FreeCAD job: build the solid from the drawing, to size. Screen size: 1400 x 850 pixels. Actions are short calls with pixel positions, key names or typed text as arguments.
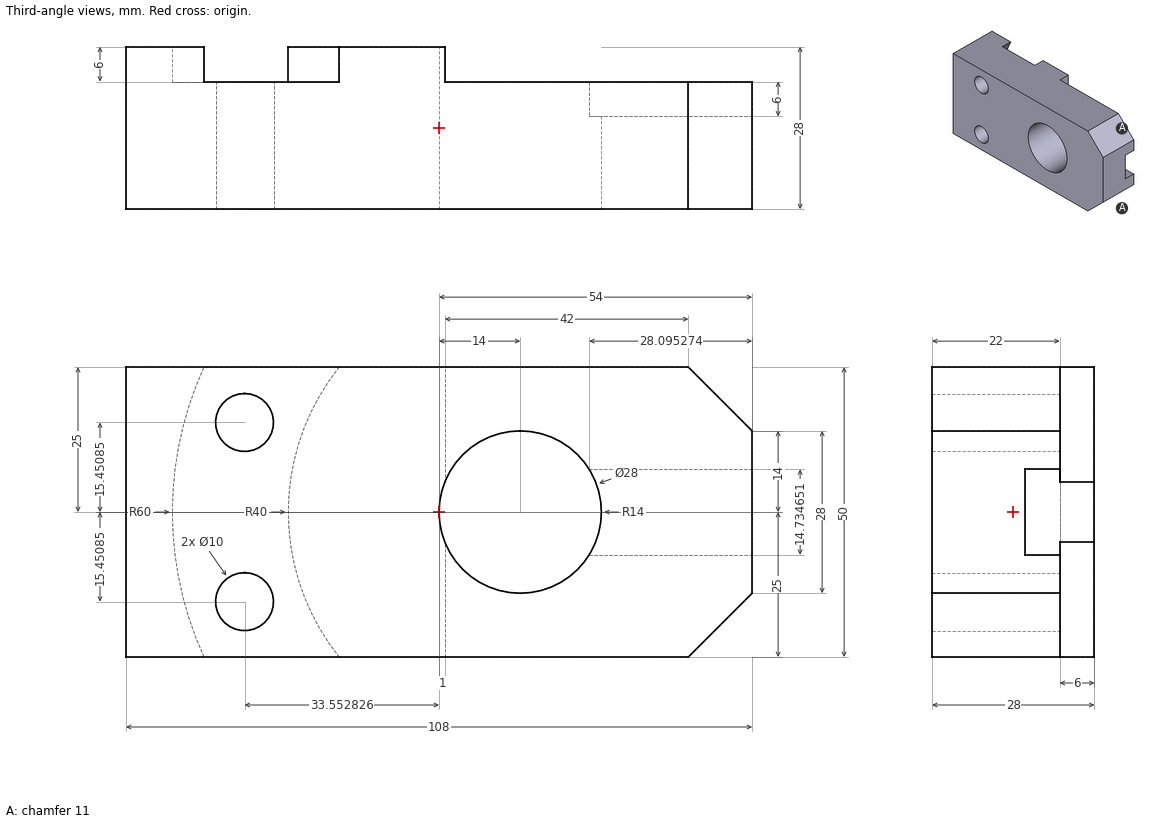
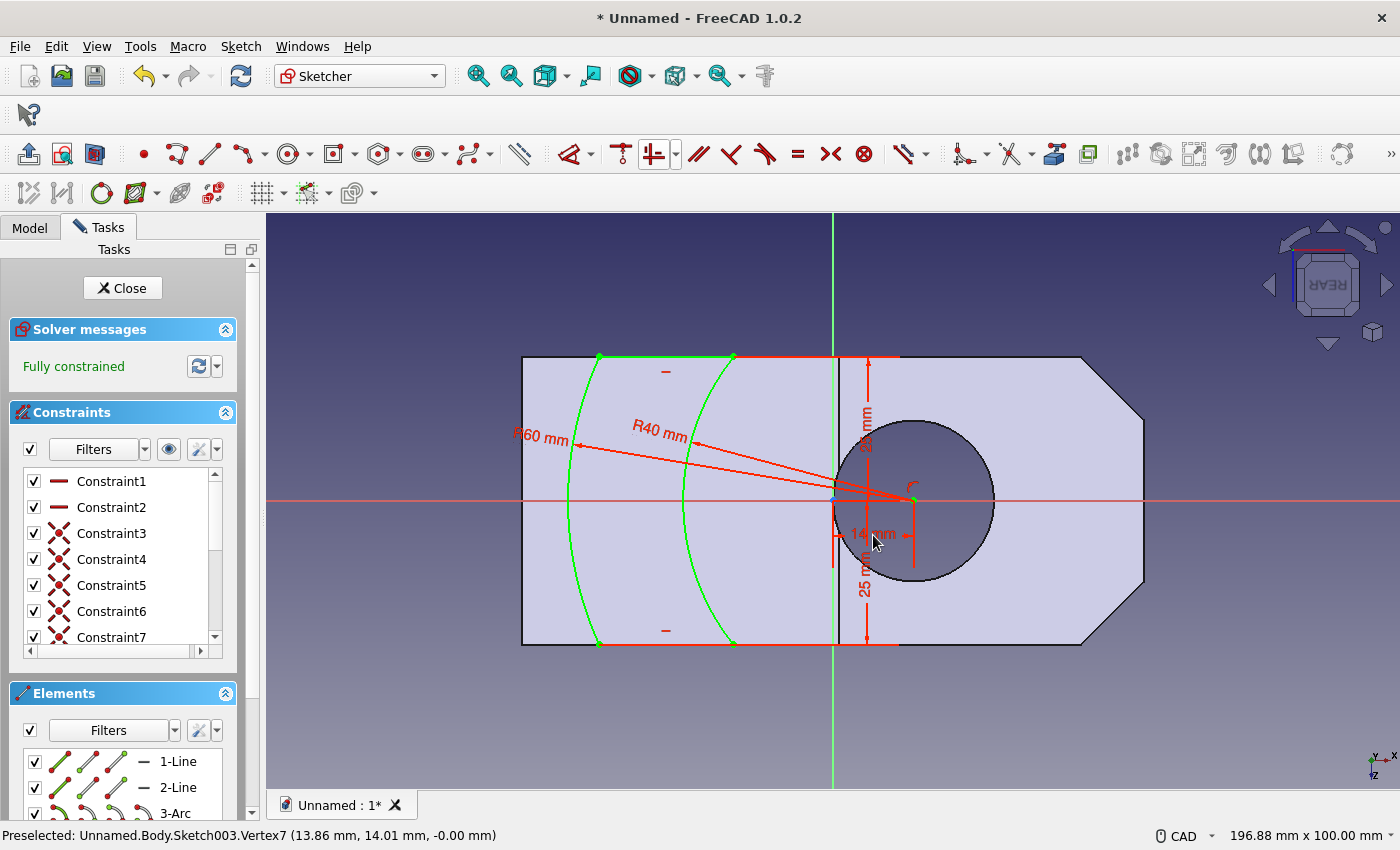
click(123, 288)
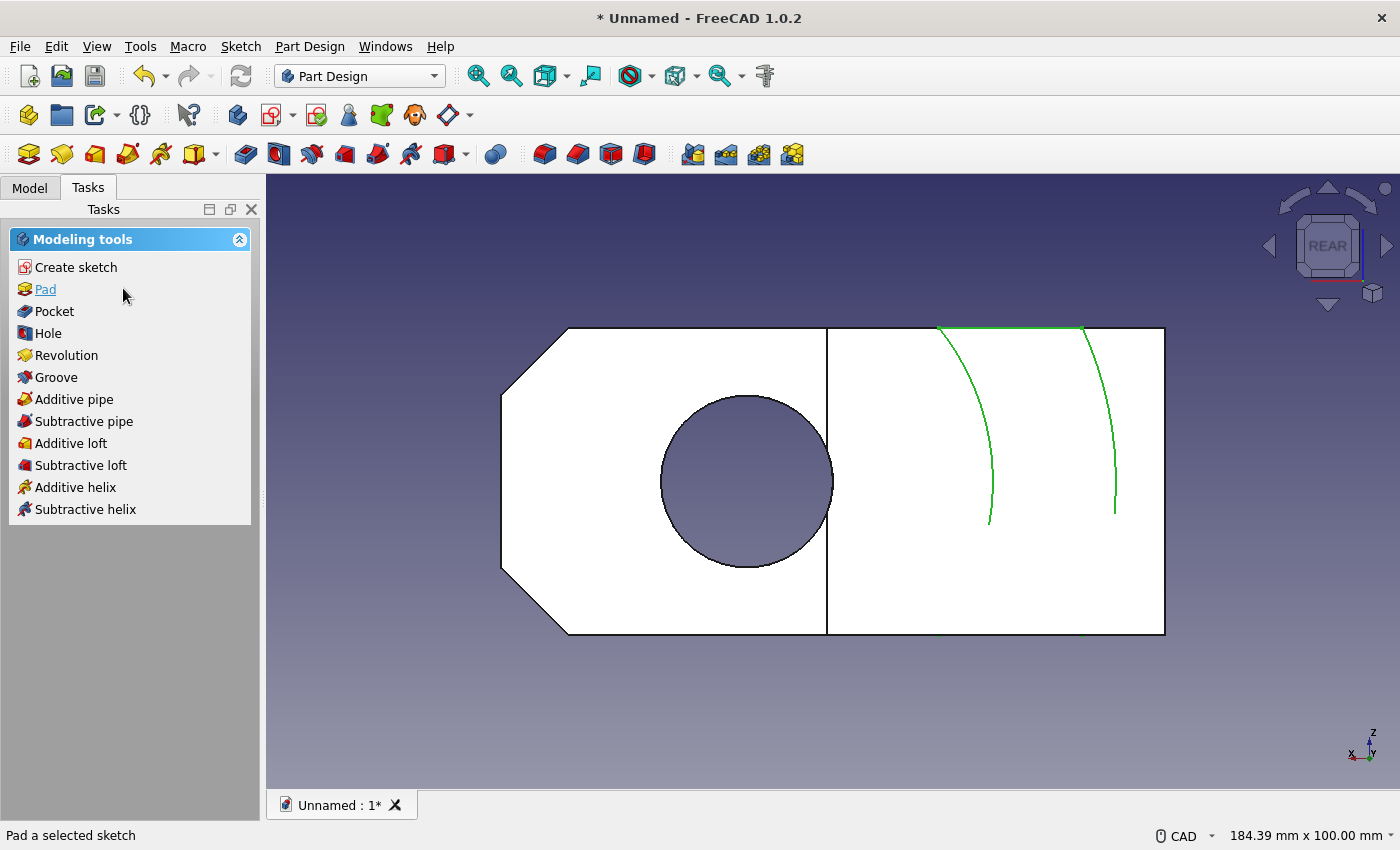
click(246, 154)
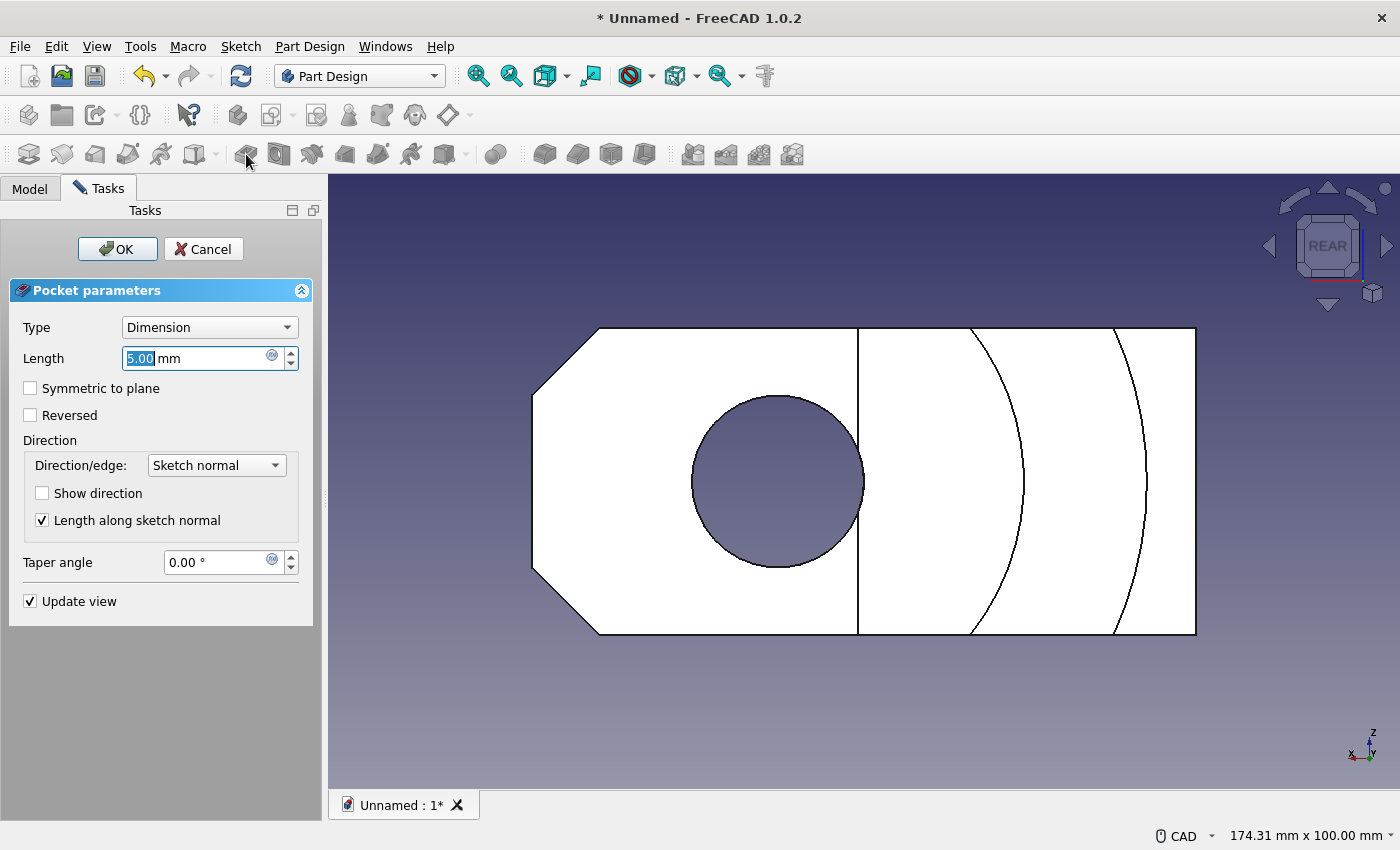
text(6)
key(Tab)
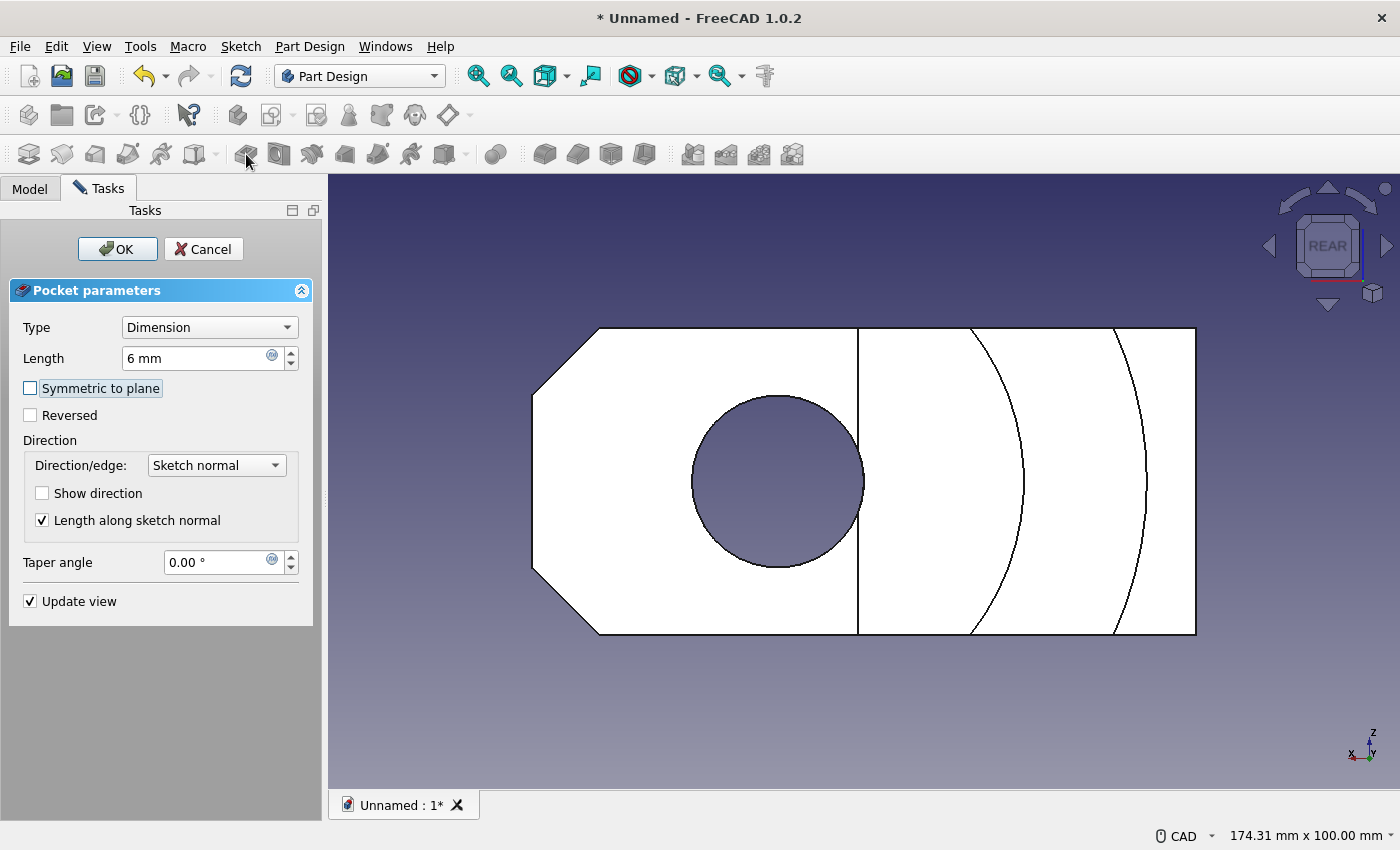
click(118, 249)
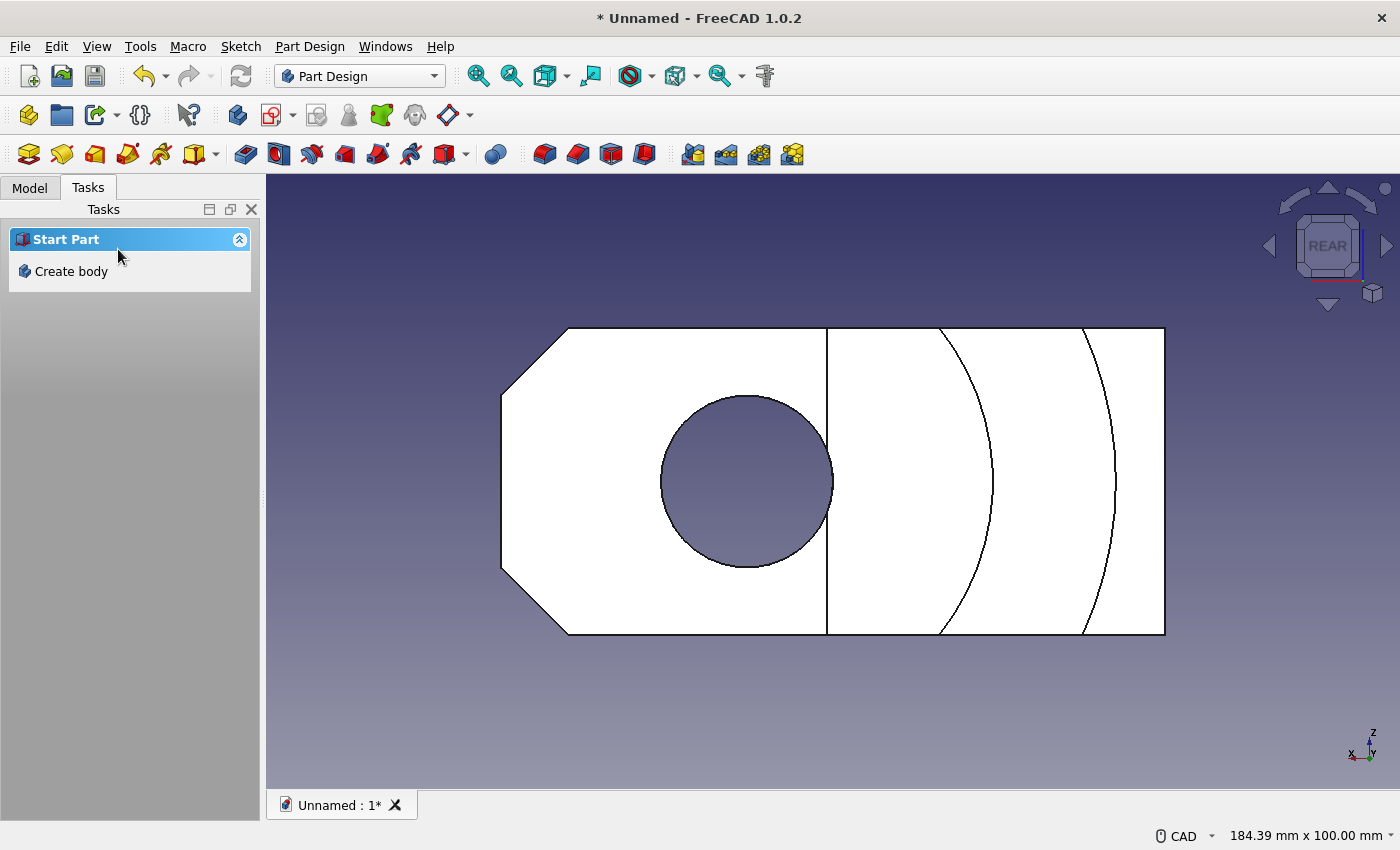
click(571, 437)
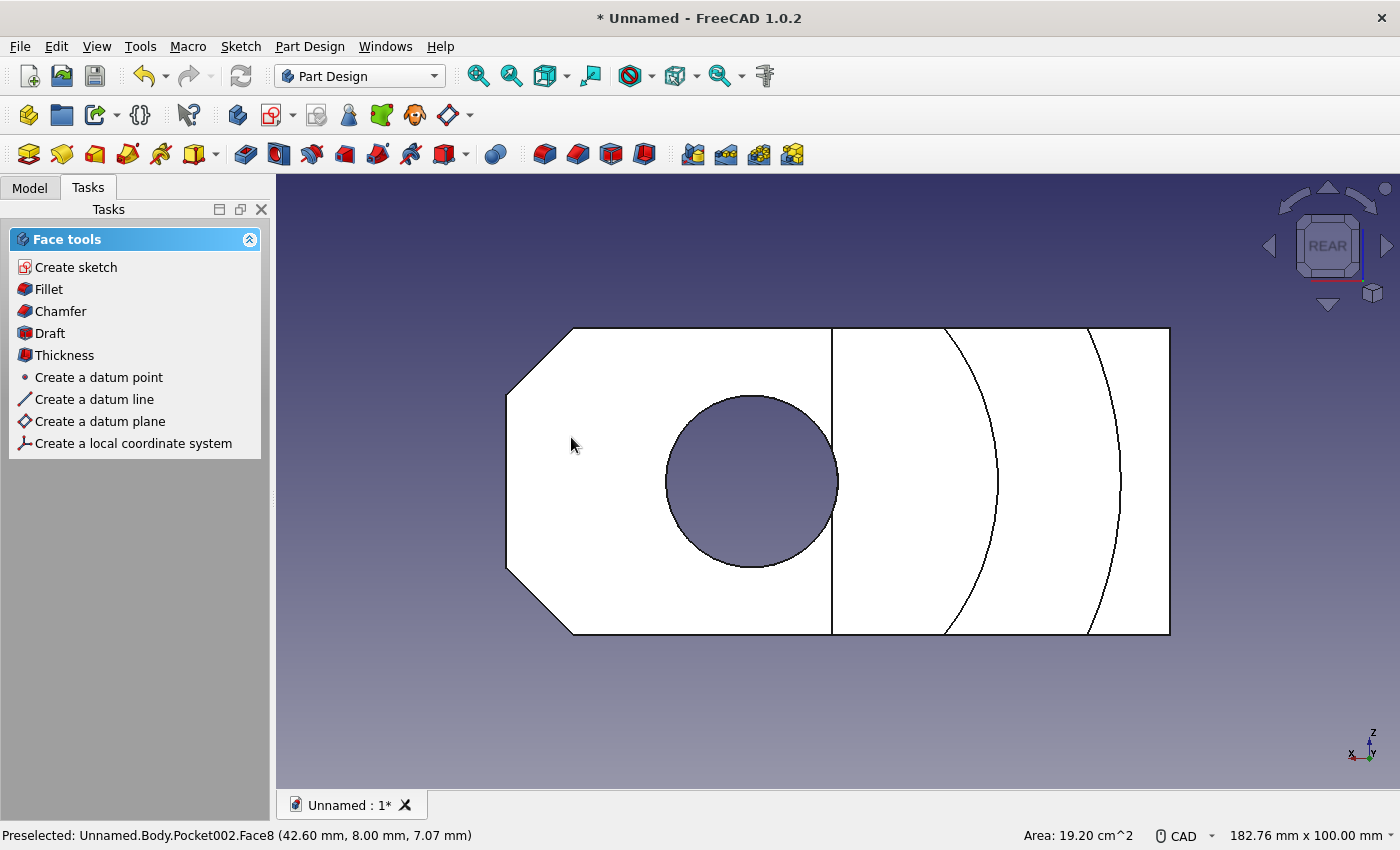
click(270, 116)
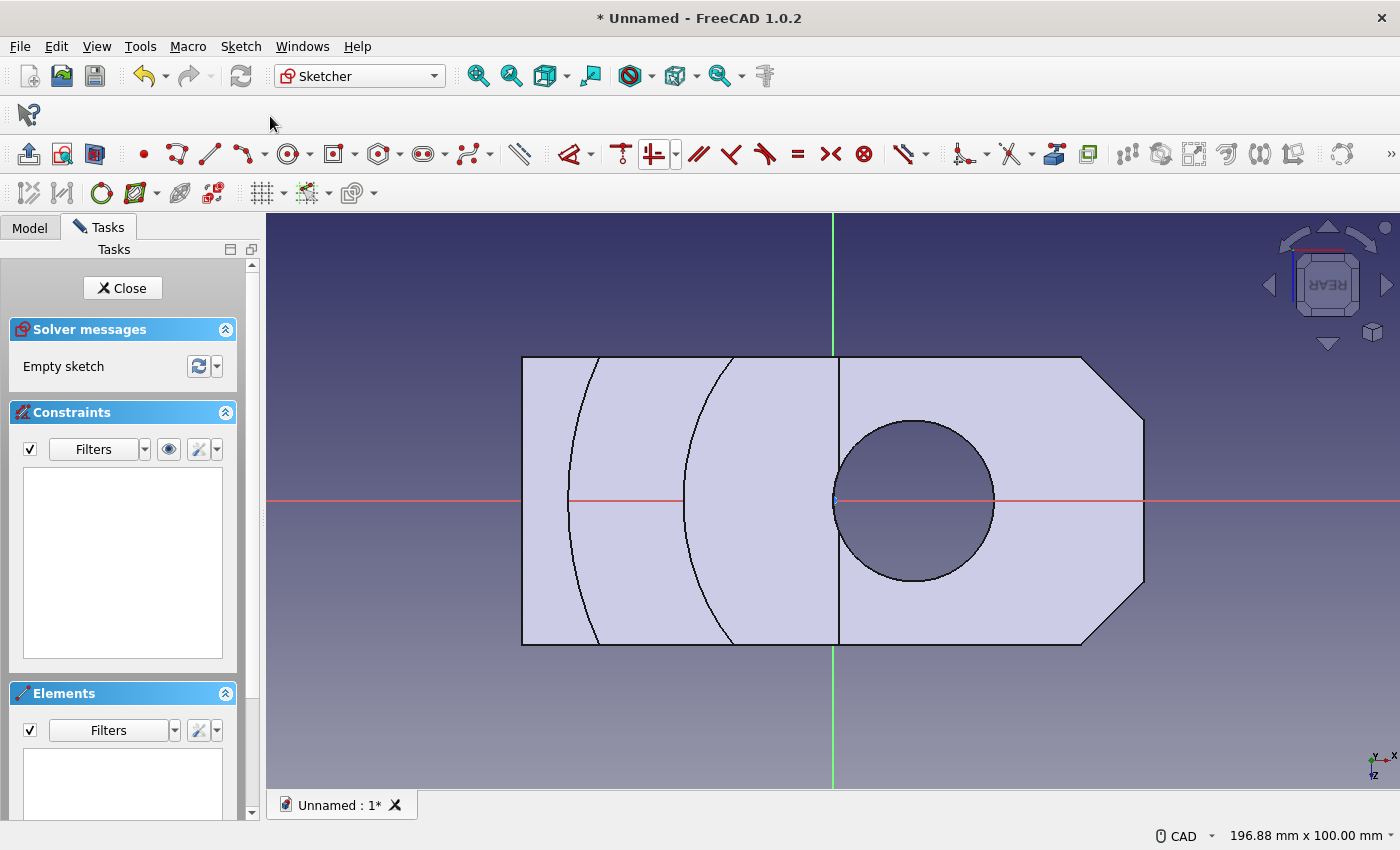
click(95, 154)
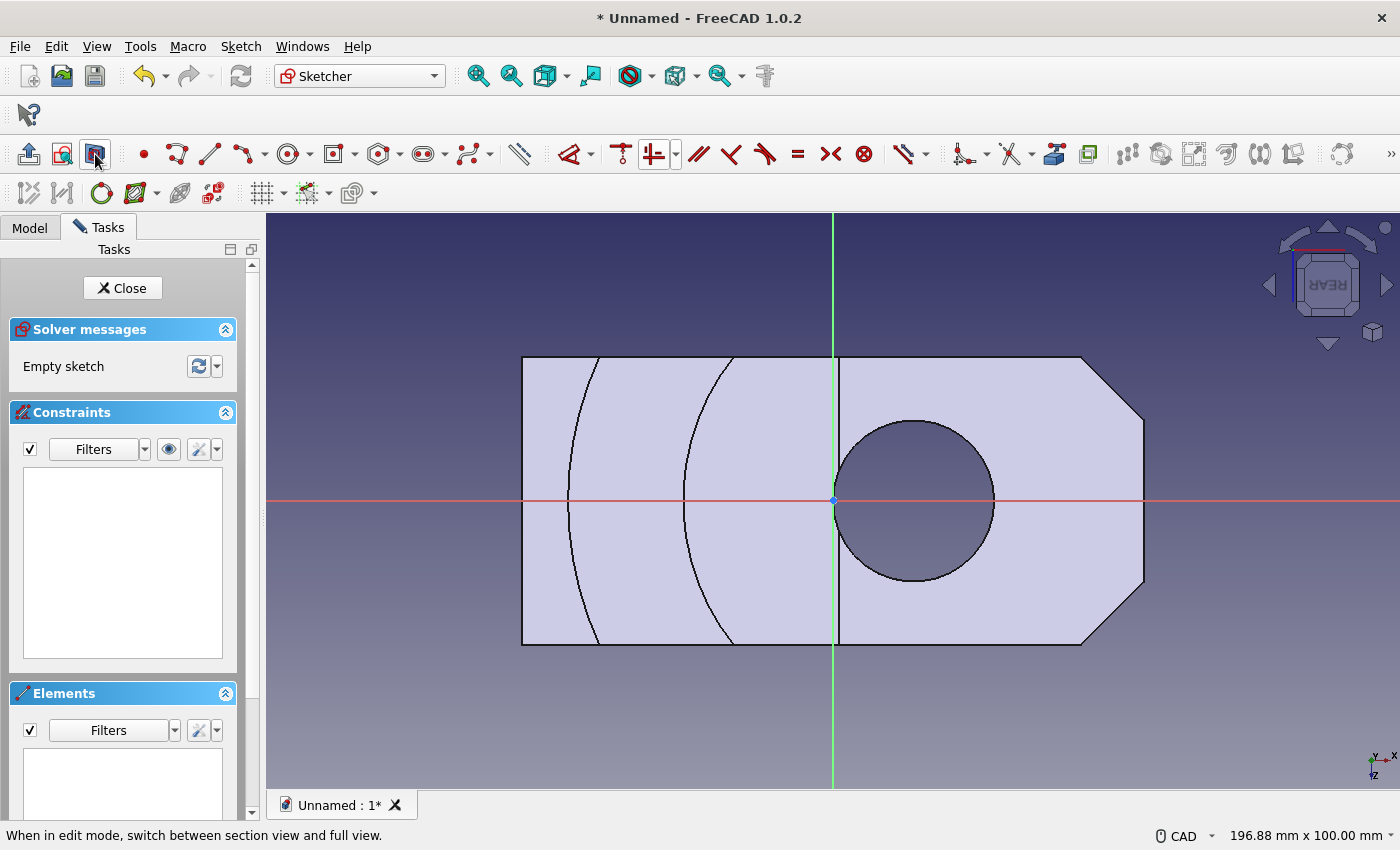
scroll(635, 501, up, 2)